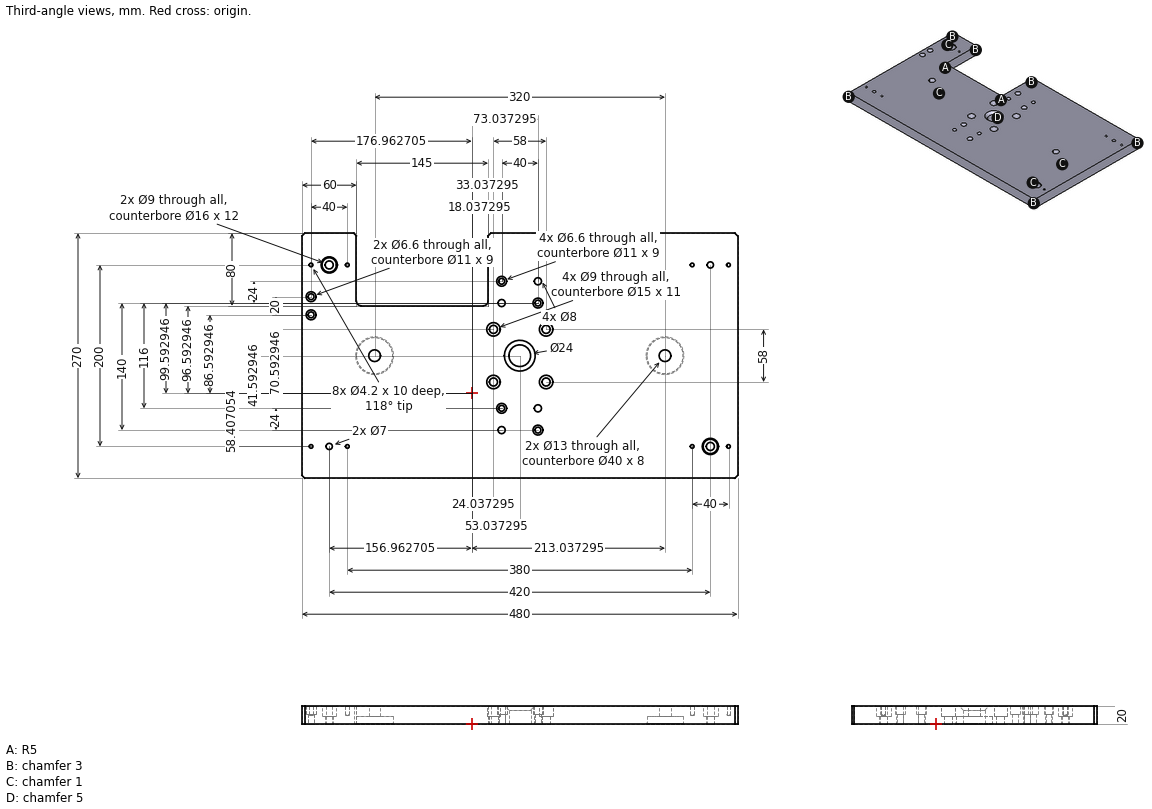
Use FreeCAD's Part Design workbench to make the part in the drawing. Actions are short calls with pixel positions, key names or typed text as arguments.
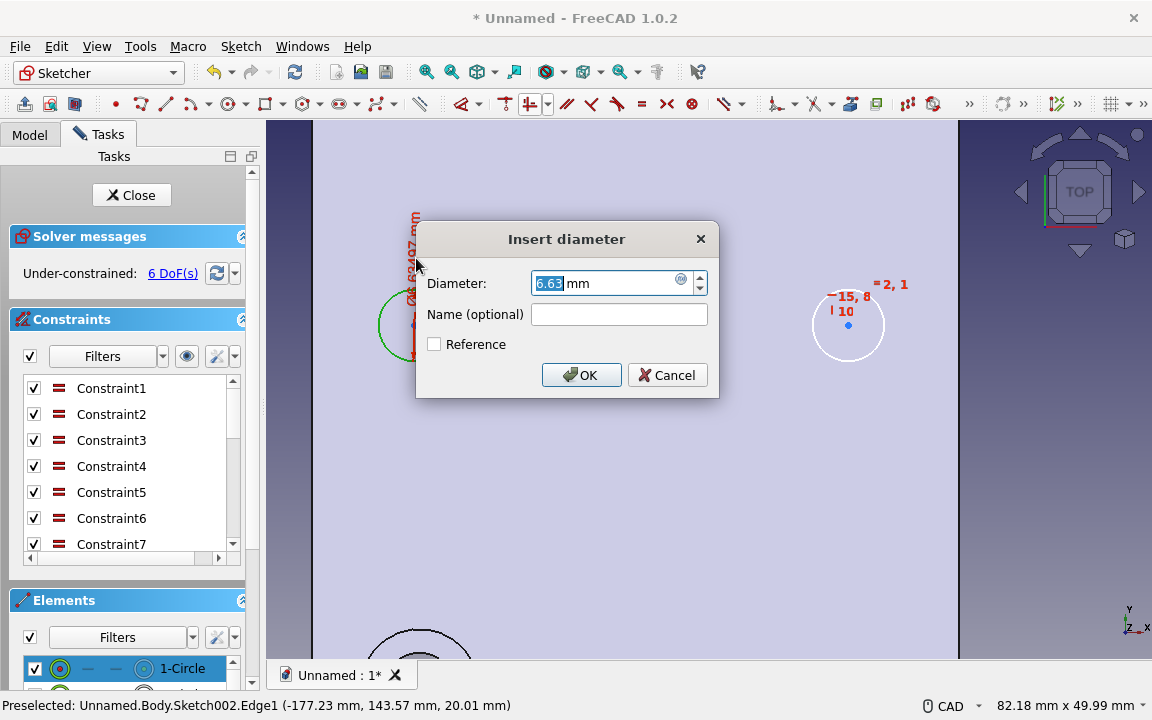
text(4.2)
key(Return)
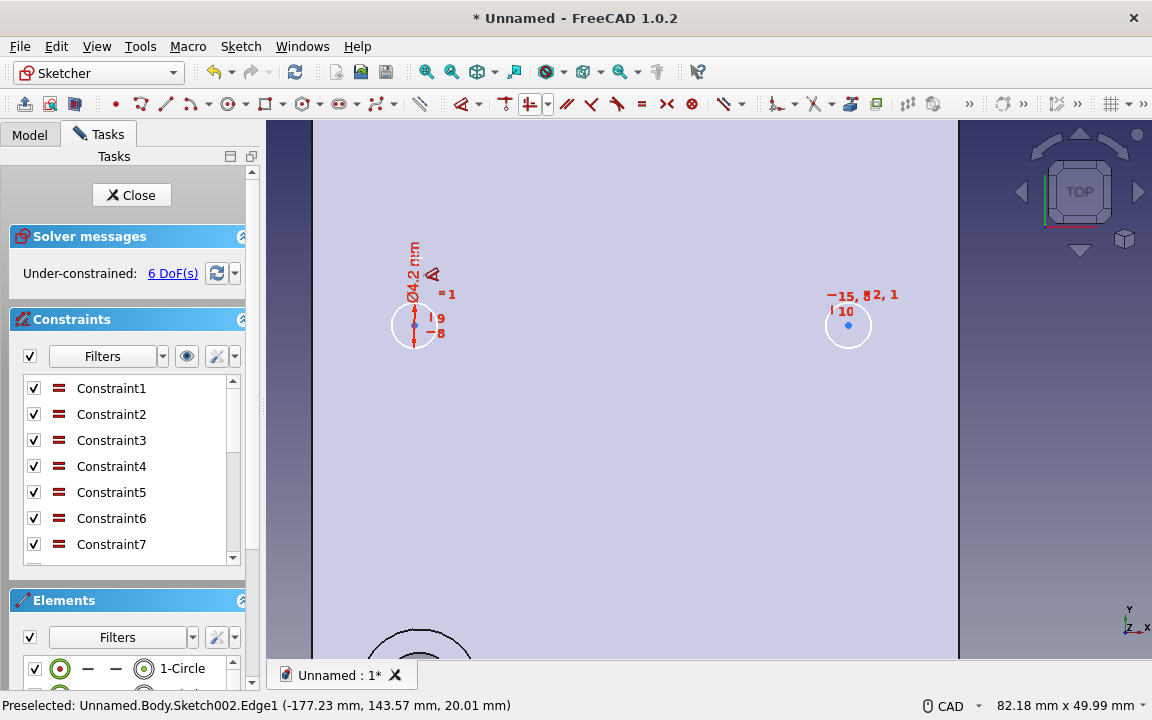
scroll(415, 290, down, 12)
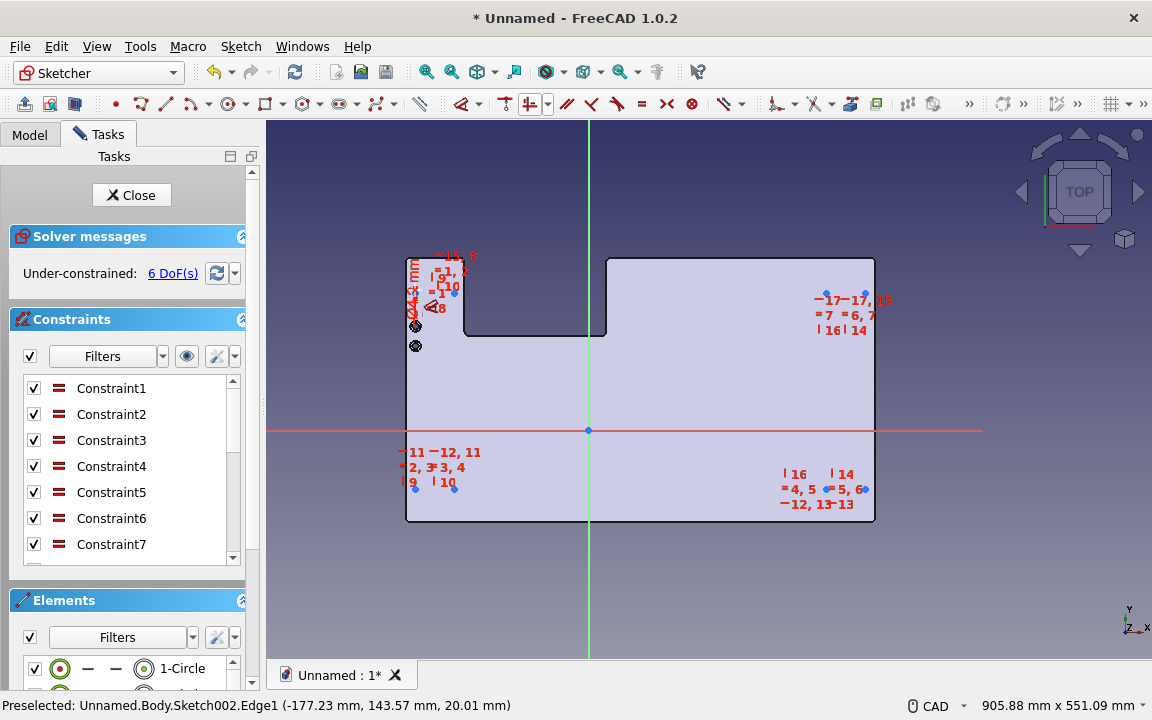
click(415, 294)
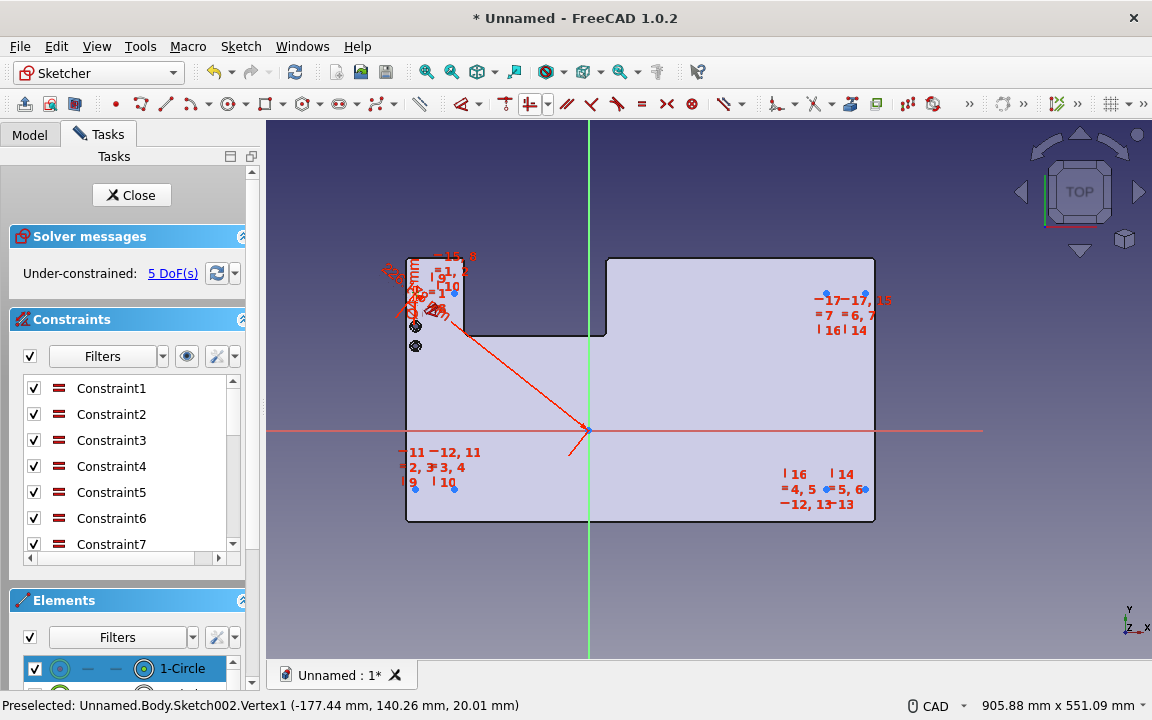
click(454, 294)
click(435, 260)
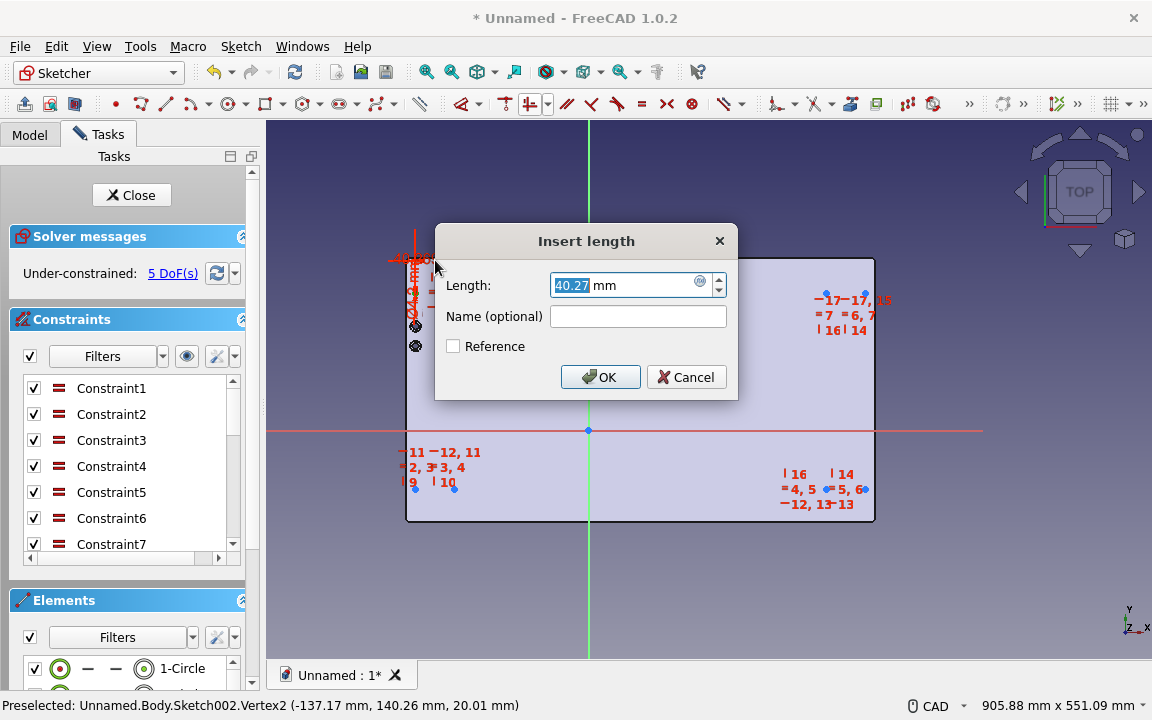
text(40)
key(Return)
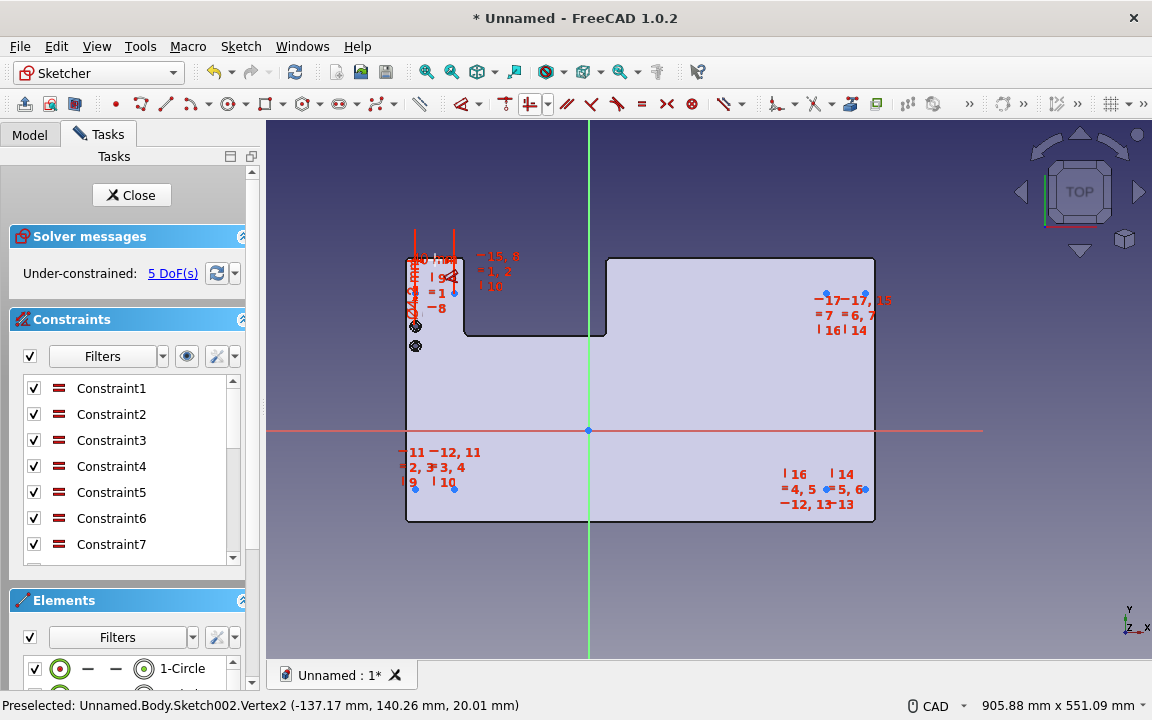
click(827, 489)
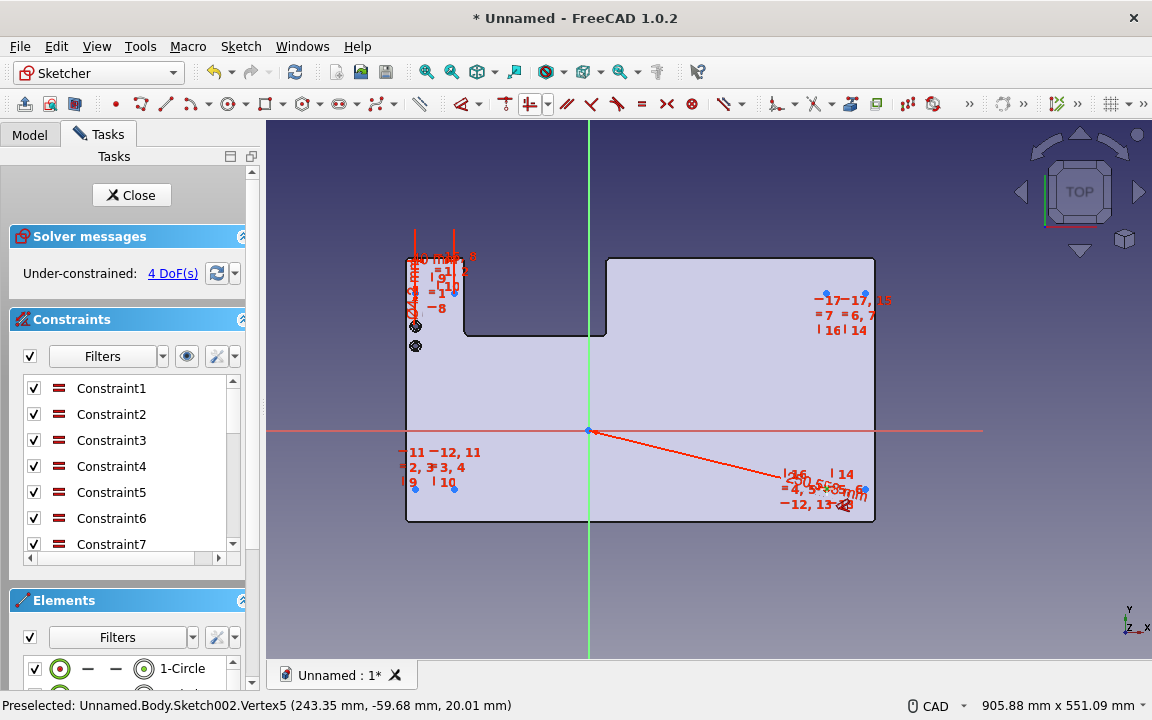
click(866, 489)
click(846, 523)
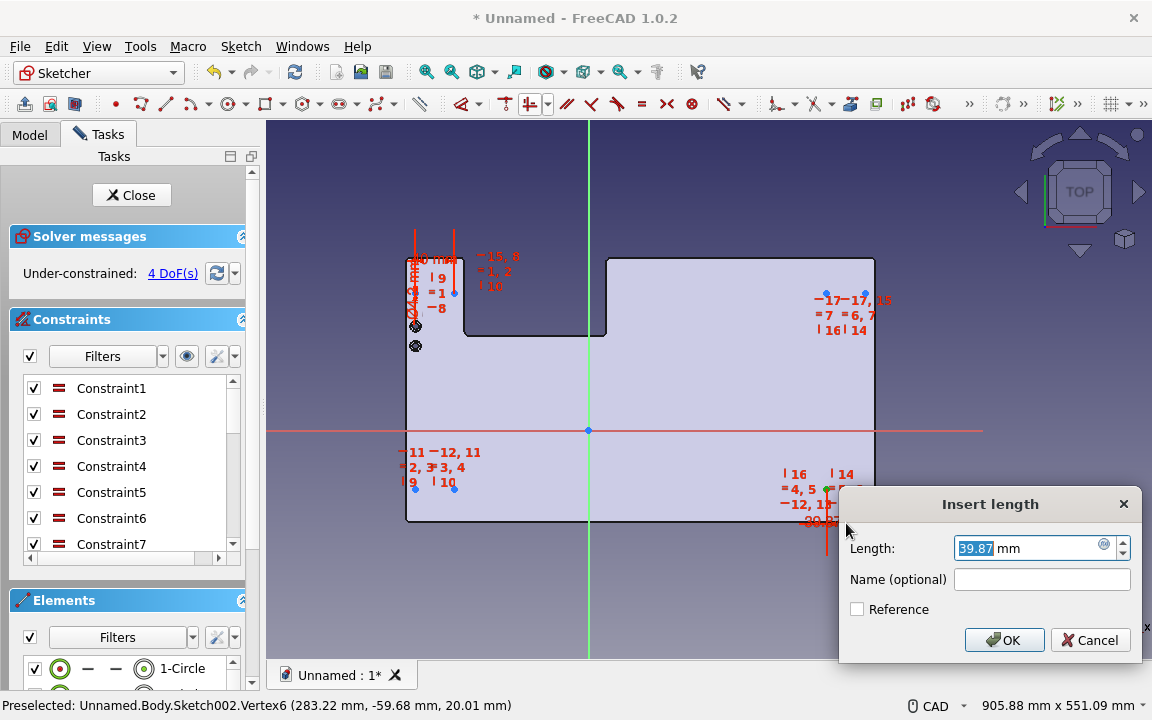
text(40)
key(Return)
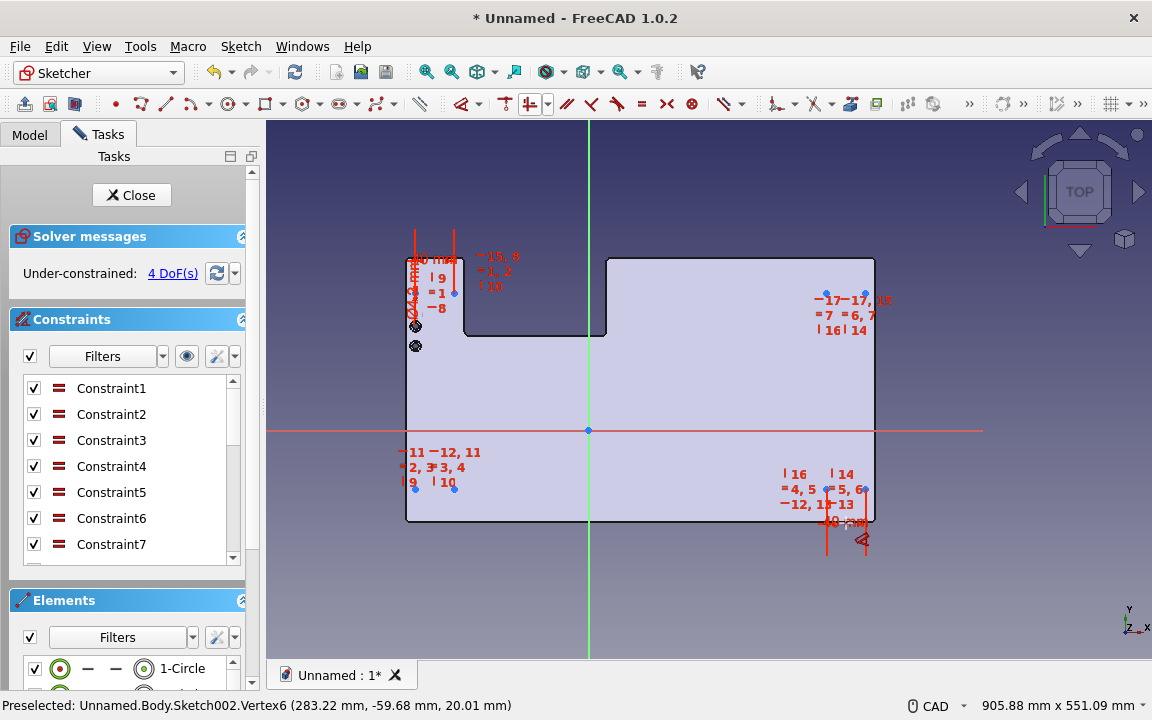
click(415, 294)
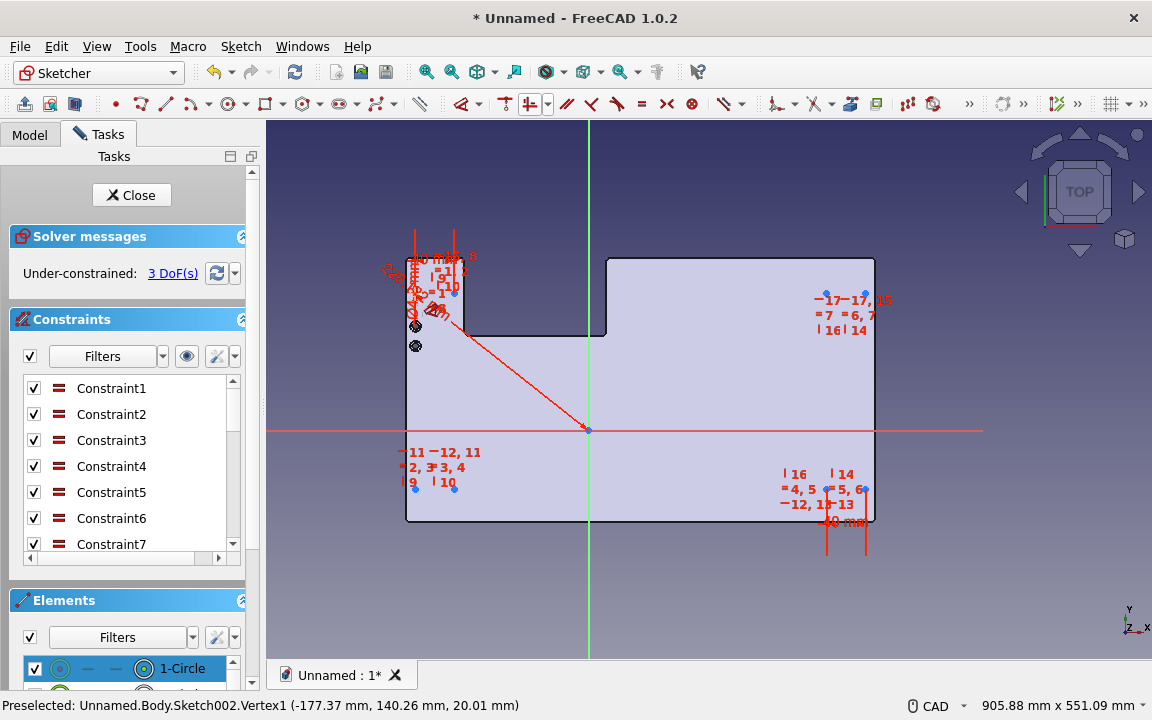
click(415, 489)
click(381, 391)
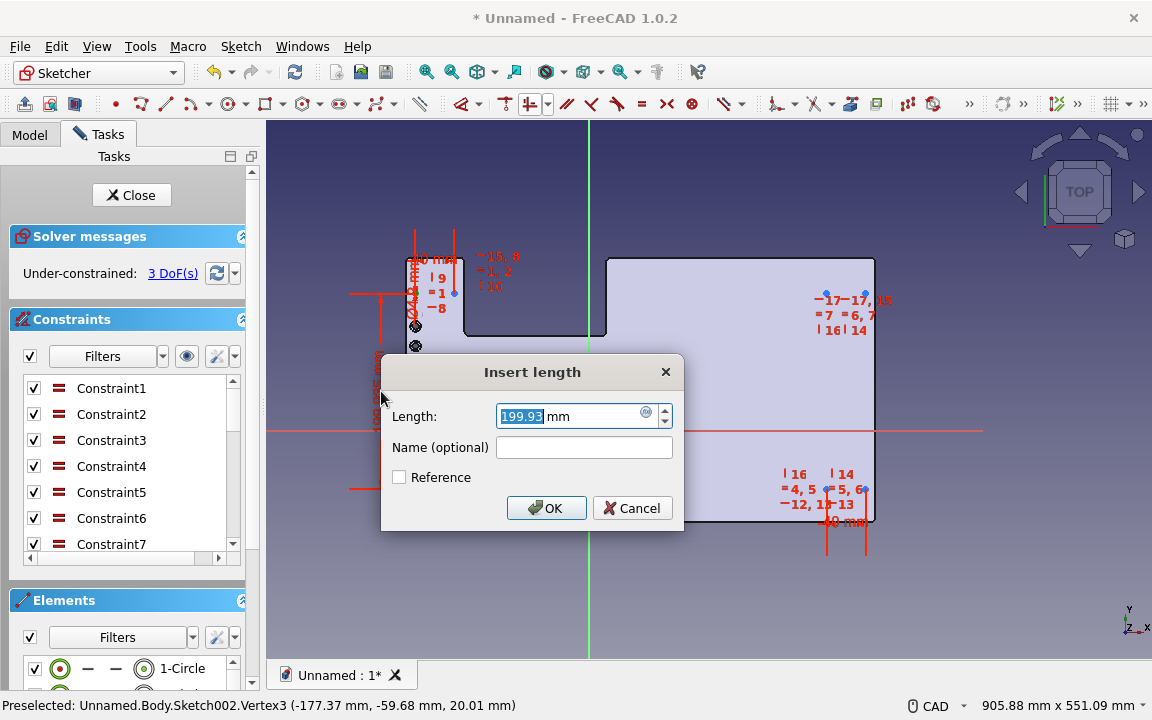
text(200)
key(Return)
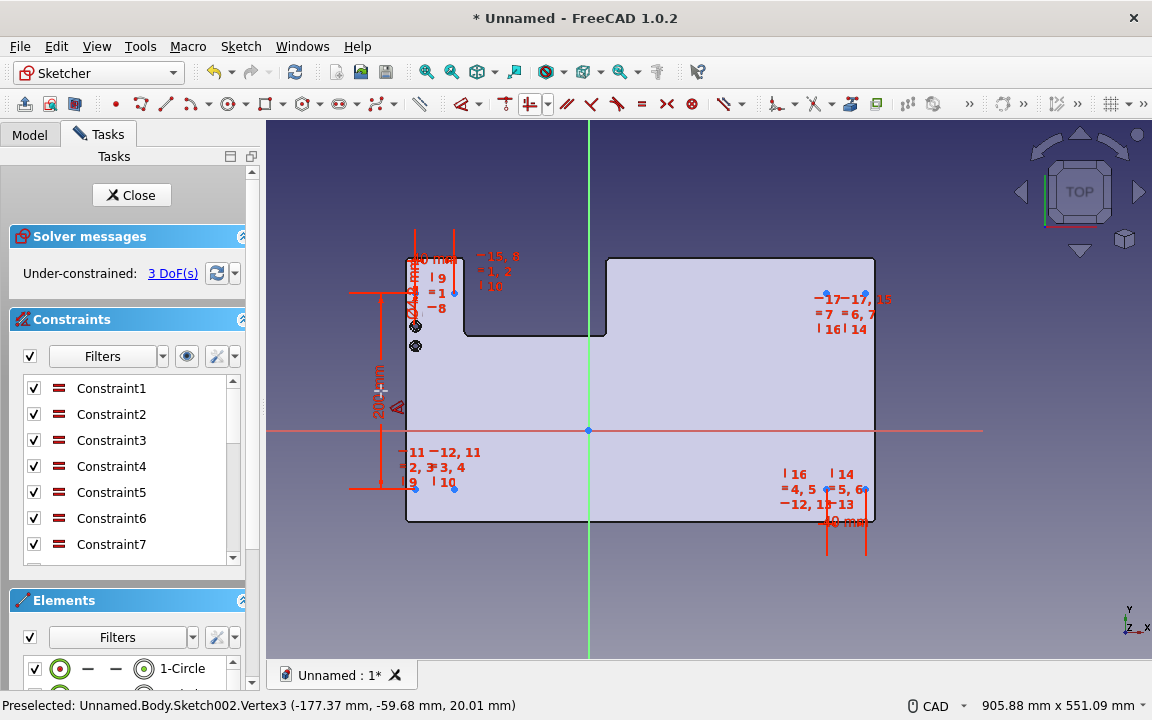
click(454, 489)